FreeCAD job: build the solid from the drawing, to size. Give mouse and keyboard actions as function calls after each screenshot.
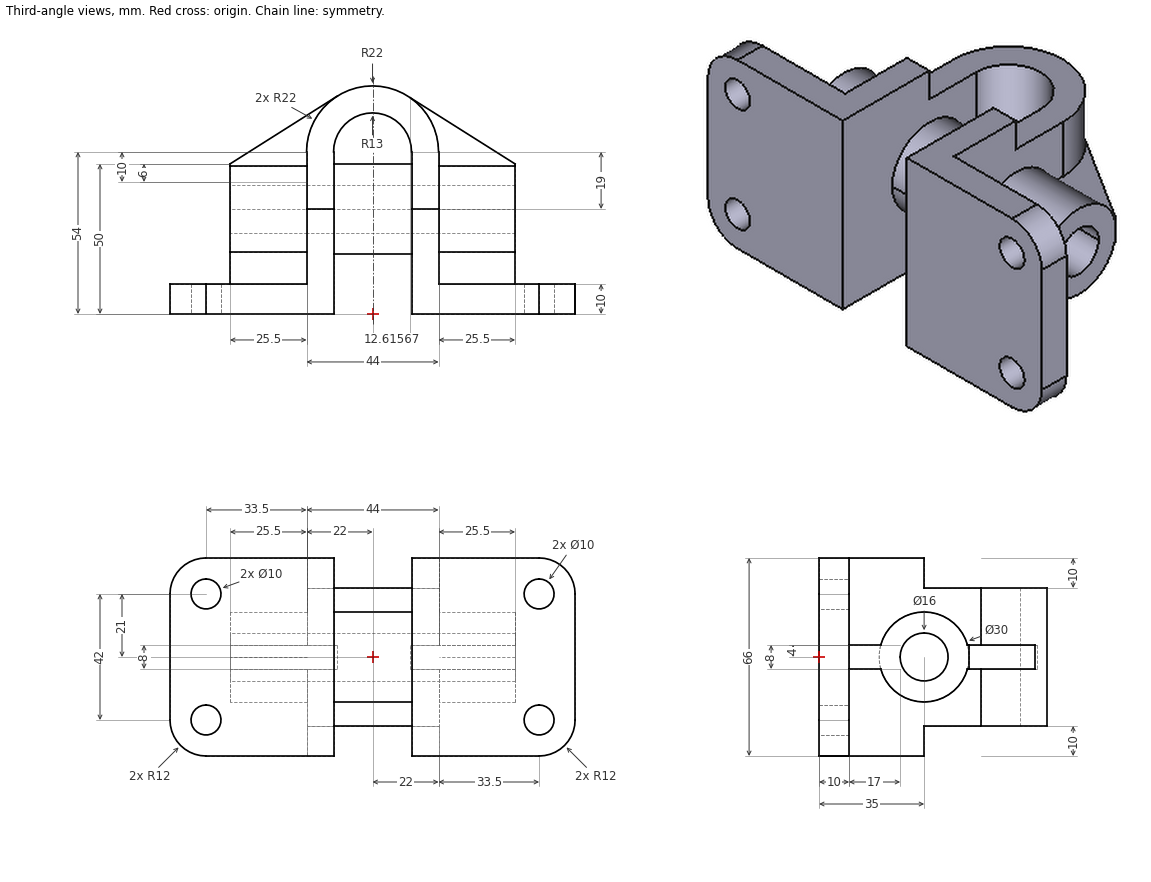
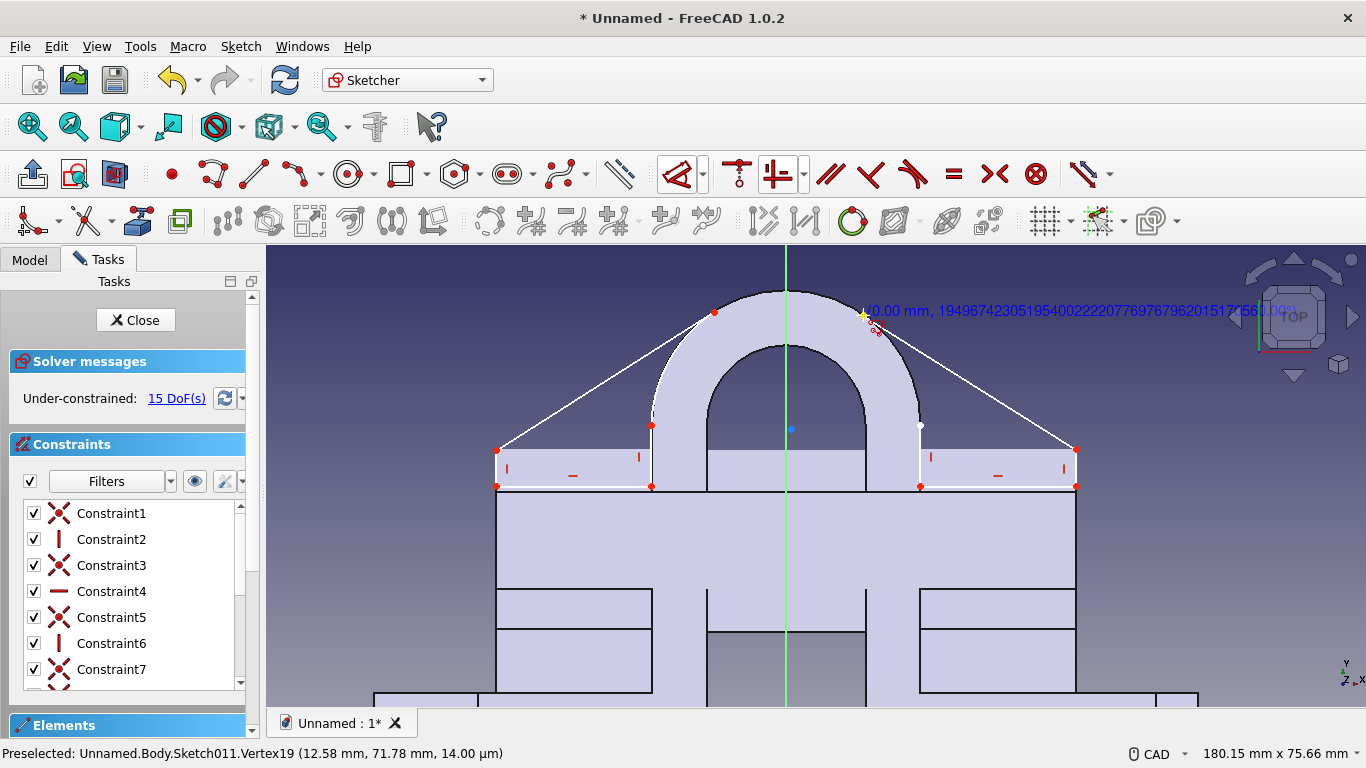
click(294, 174)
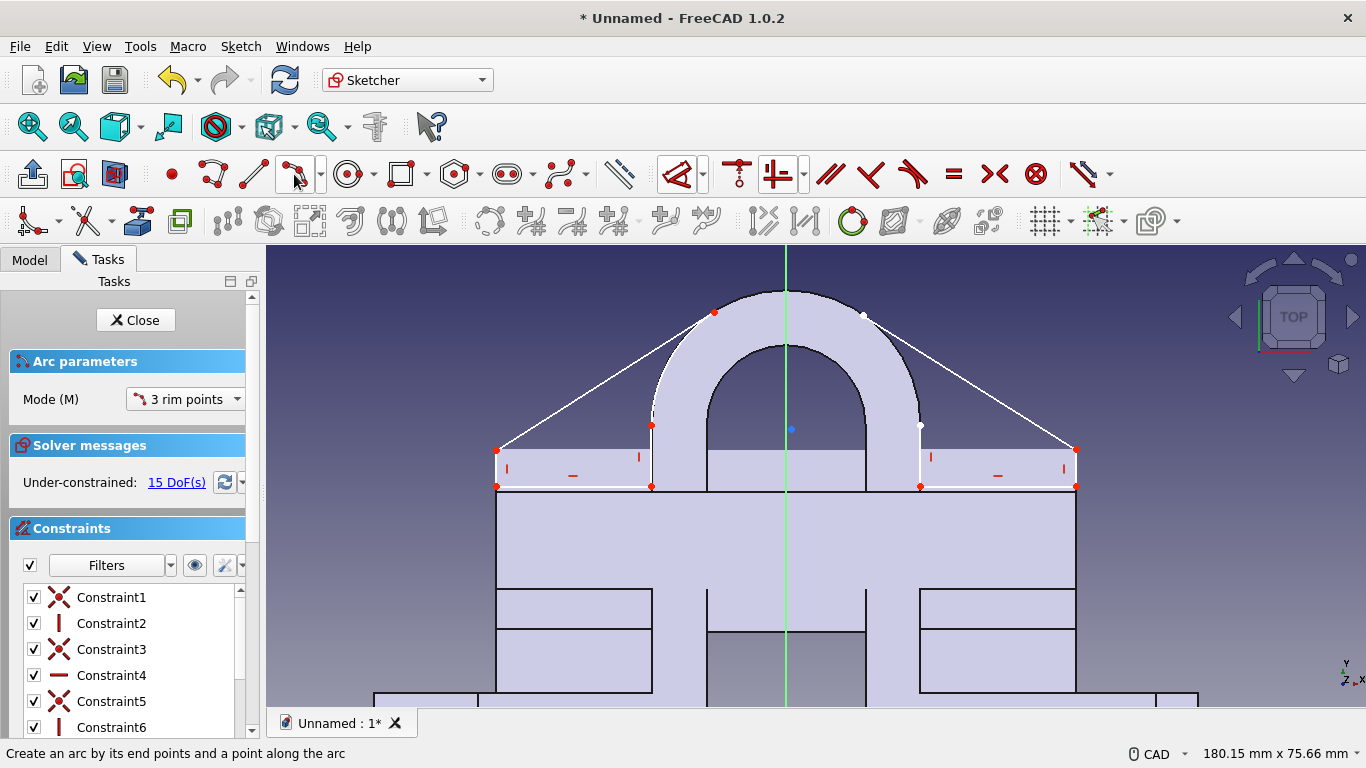
click(863, 316)
click(920, 426)
click(905, 363)
key(Escape)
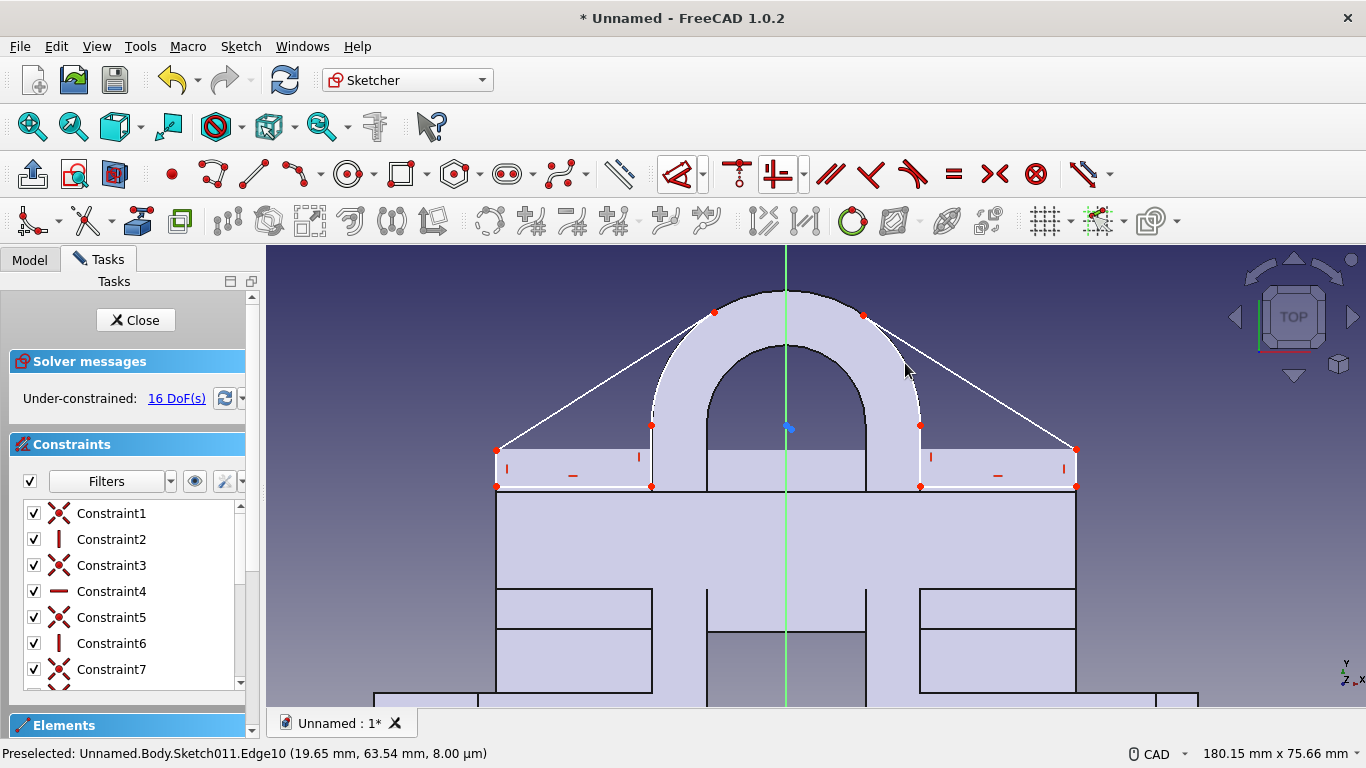
click(649, 354)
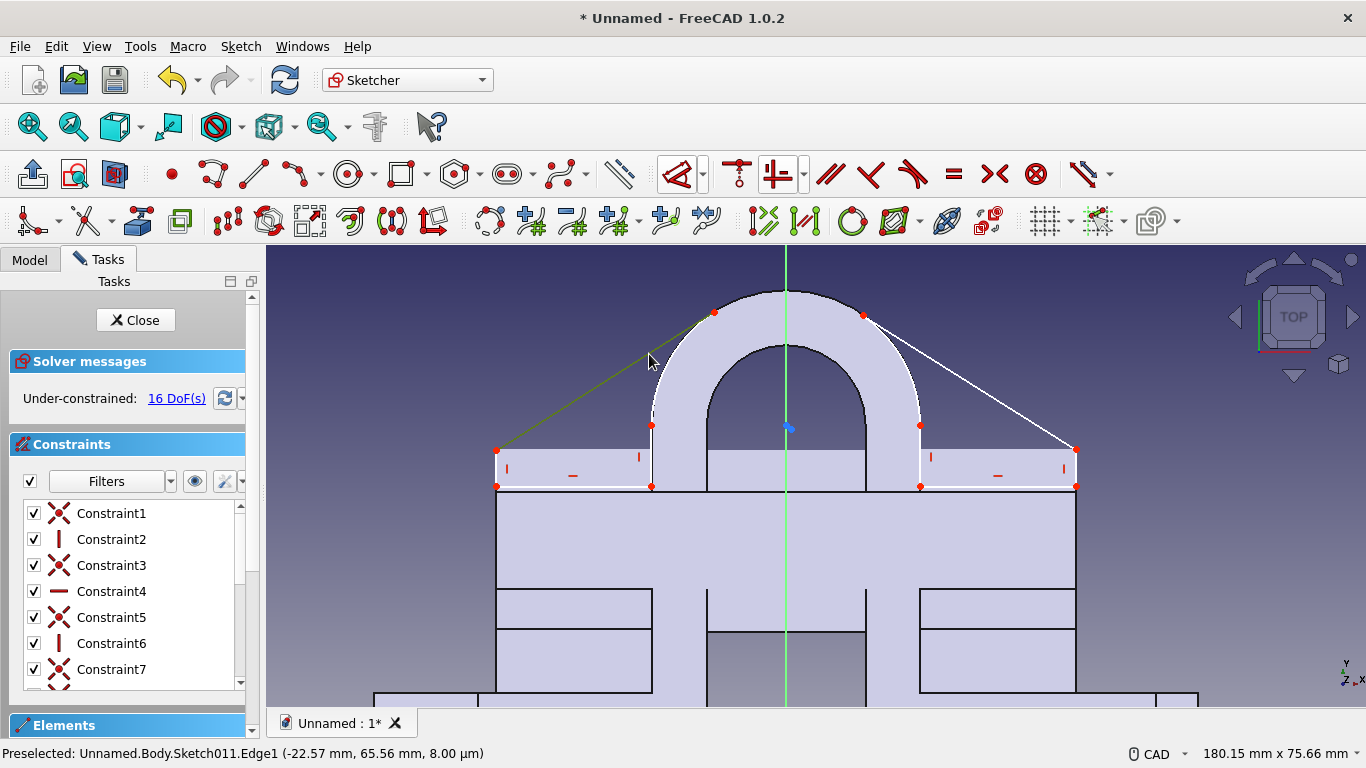
click(658, 386)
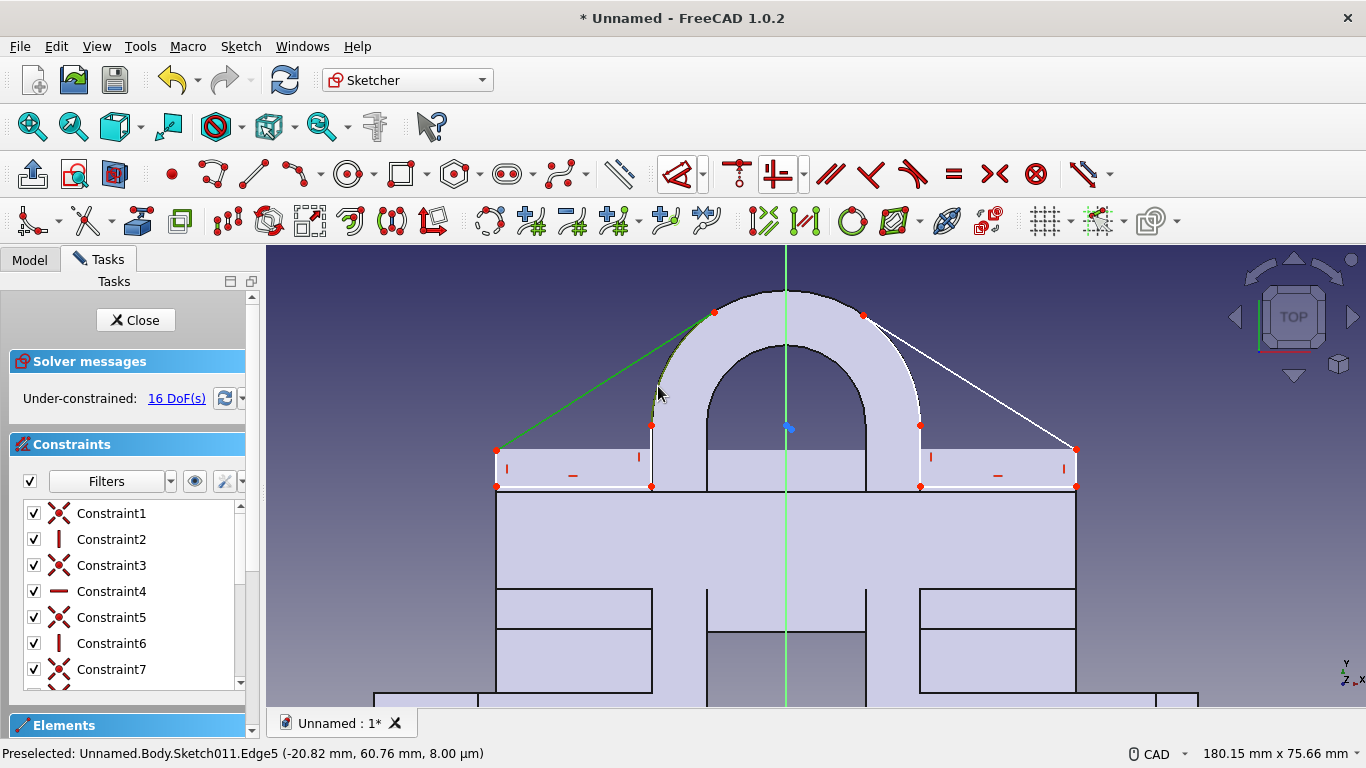
click(913, 174)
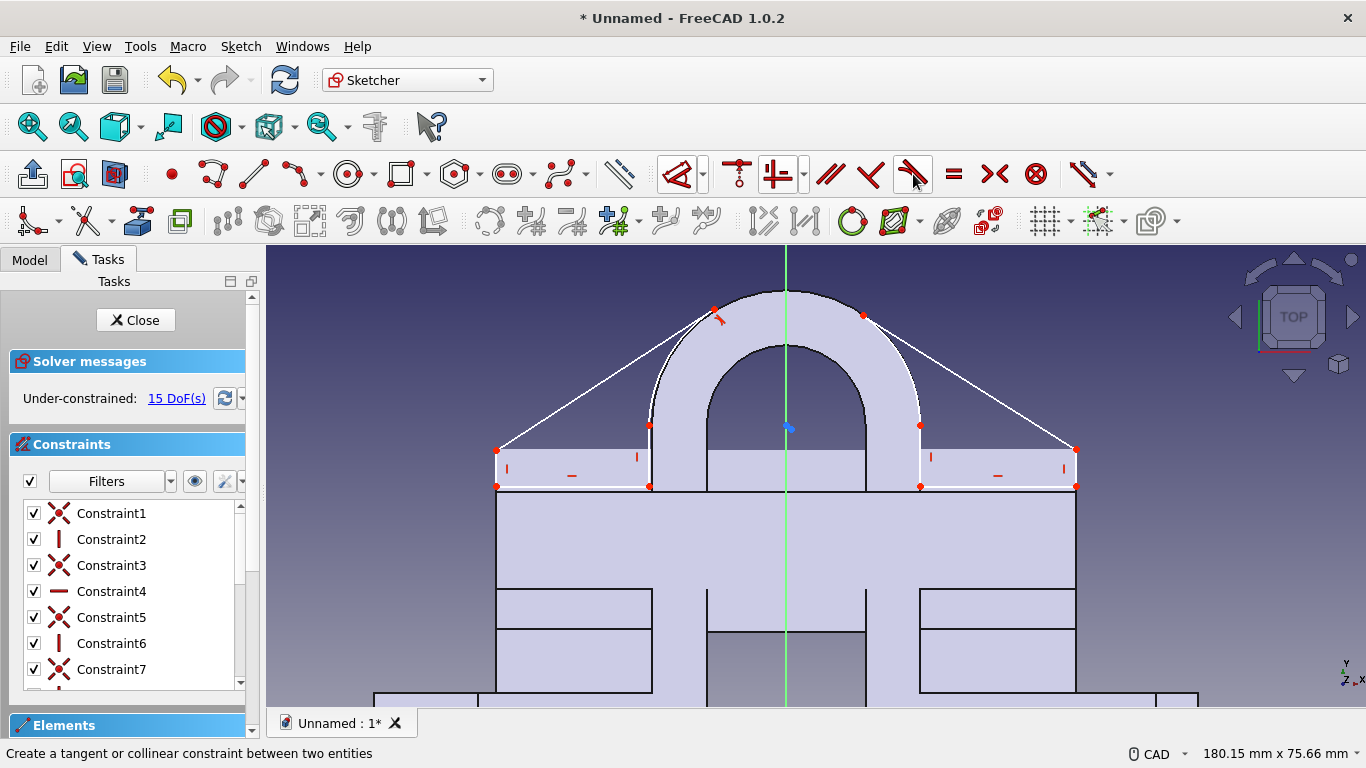
click(649, 468)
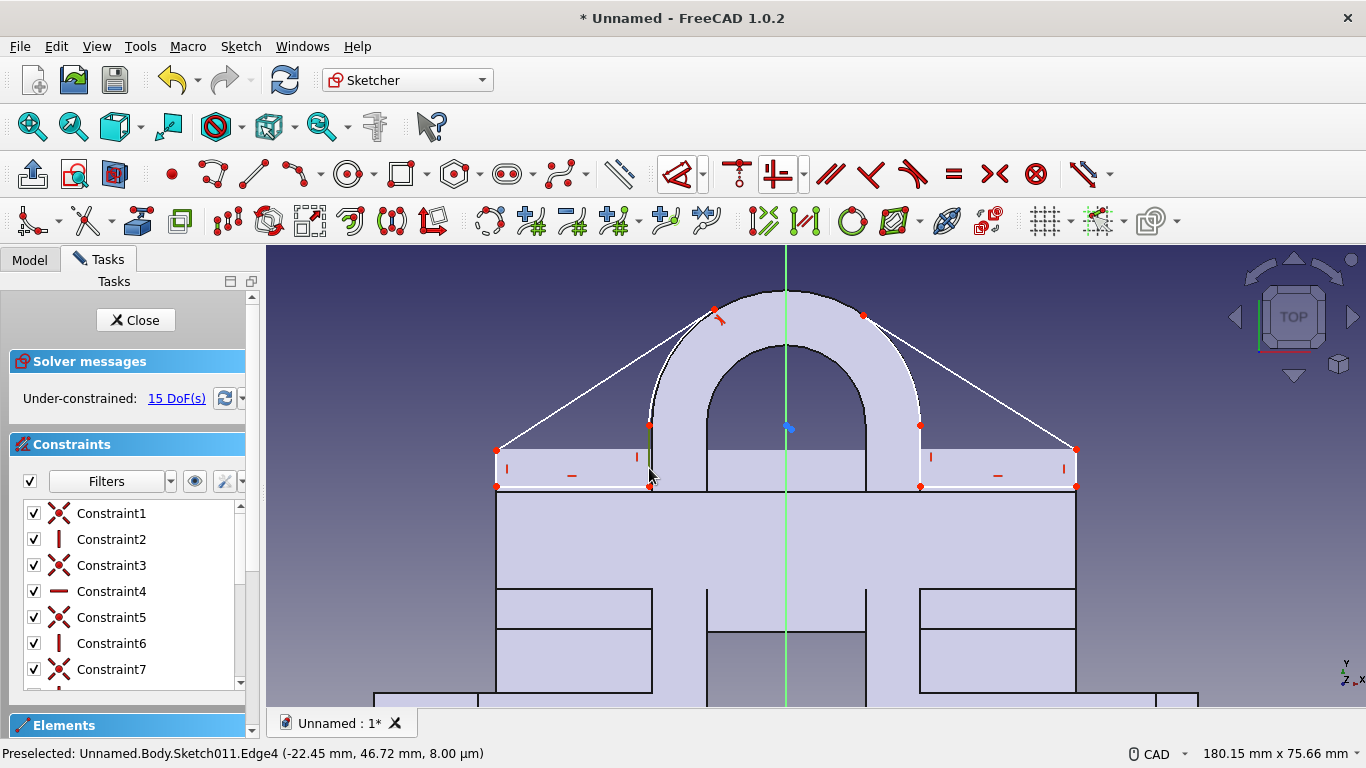
click(656, 385)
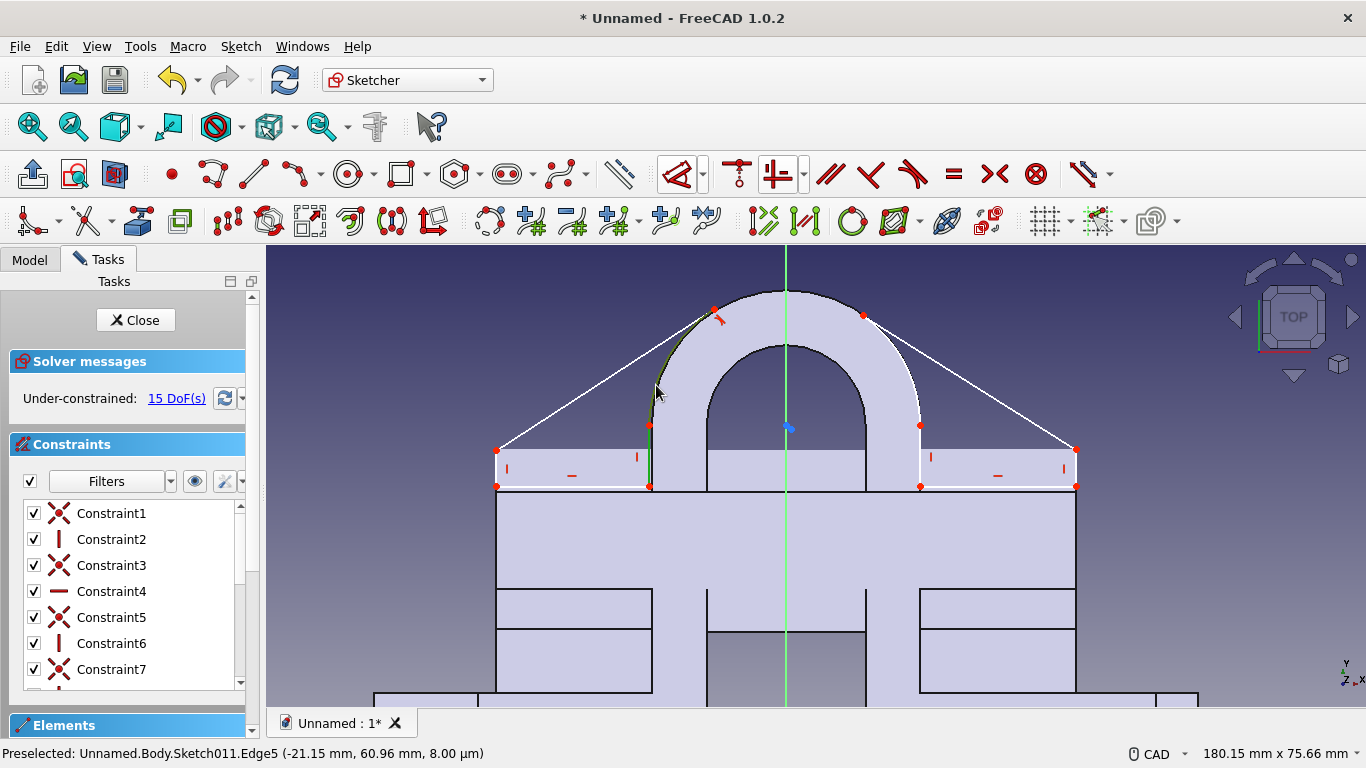
click(913, 174)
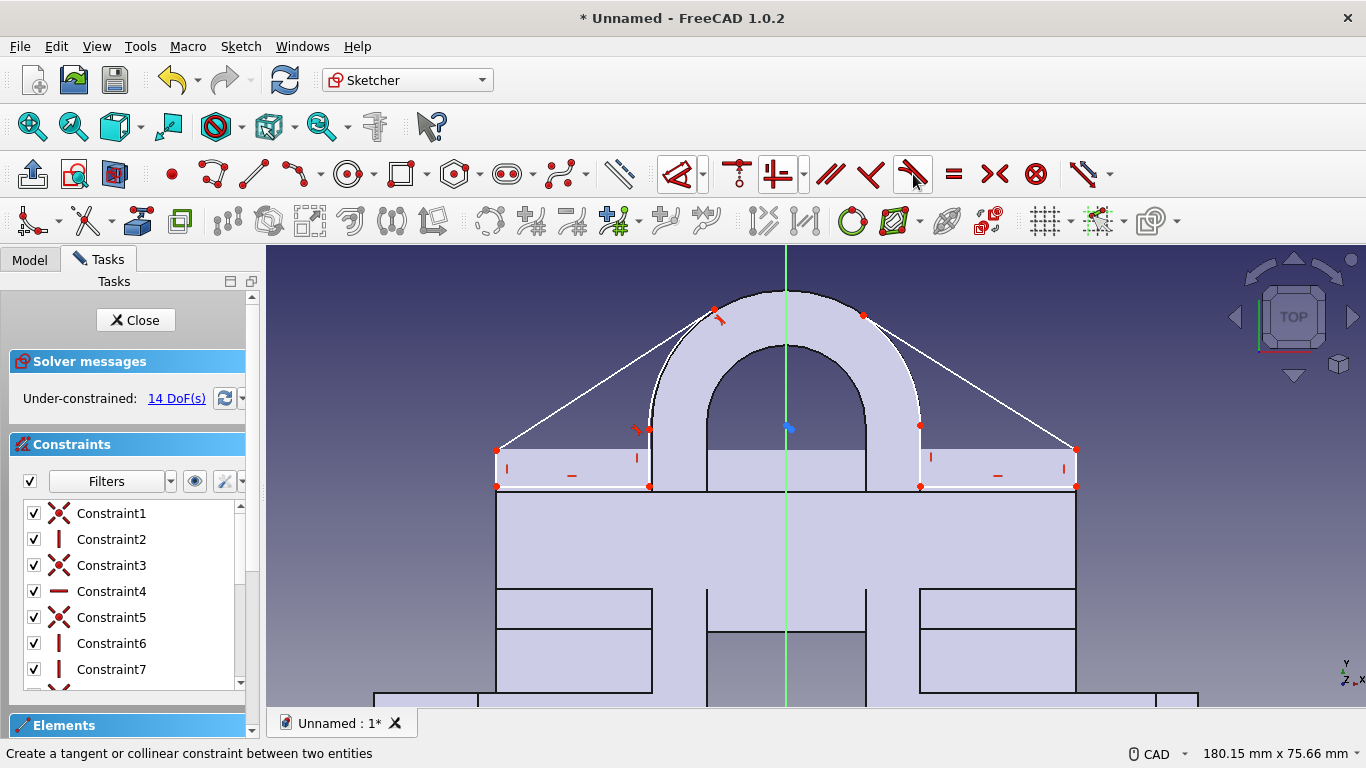
click(920, 444)